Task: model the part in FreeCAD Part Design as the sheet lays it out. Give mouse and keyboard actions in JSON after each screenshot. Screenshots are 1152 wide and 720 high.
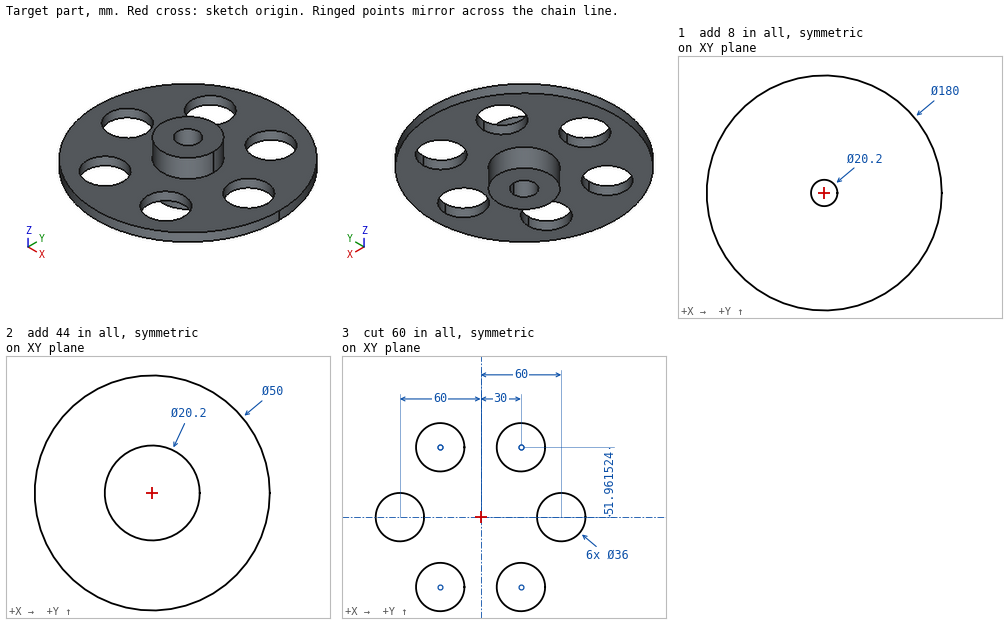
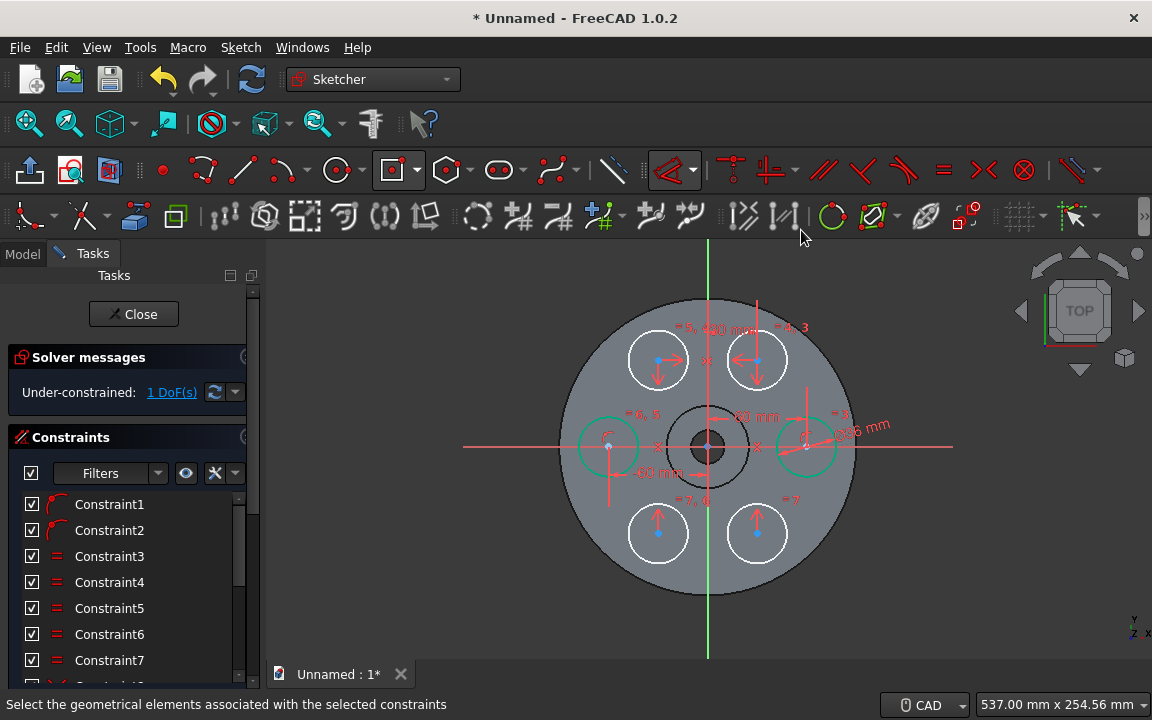
{"action": "left_click", "coordinate": [757, 360]}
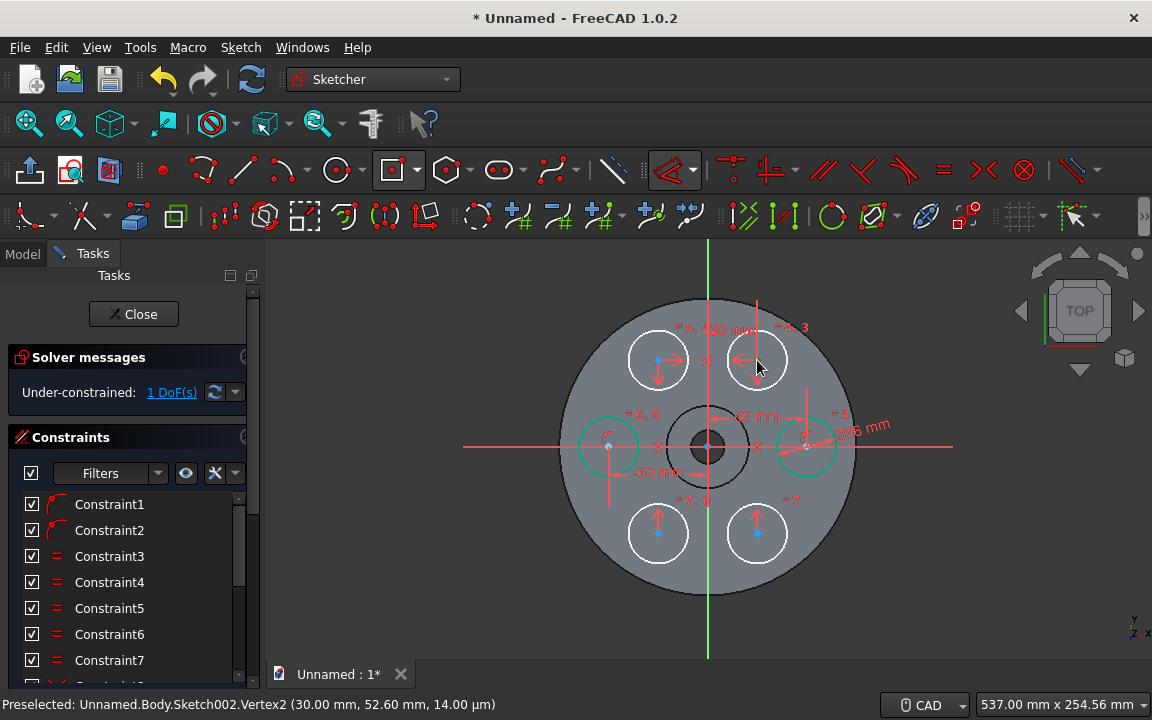
{"action": "key", "text": "i"}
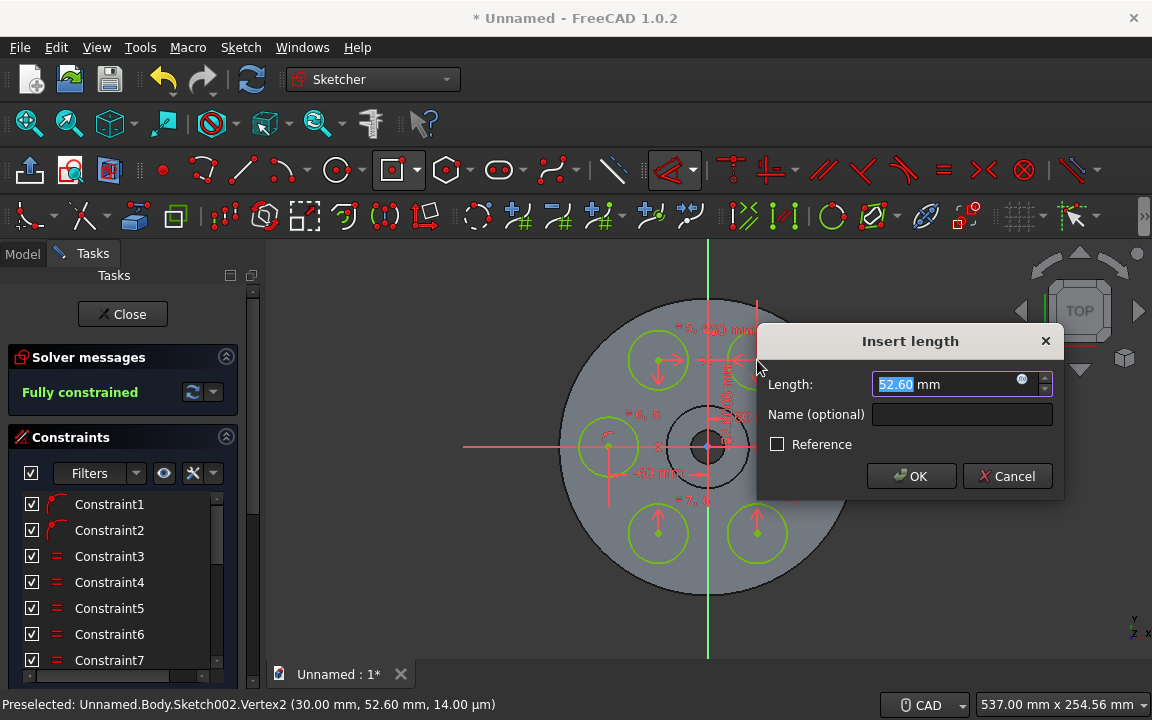
{"action": "type", "text": "51.961524"}
{"action": "key", "text": "Return"}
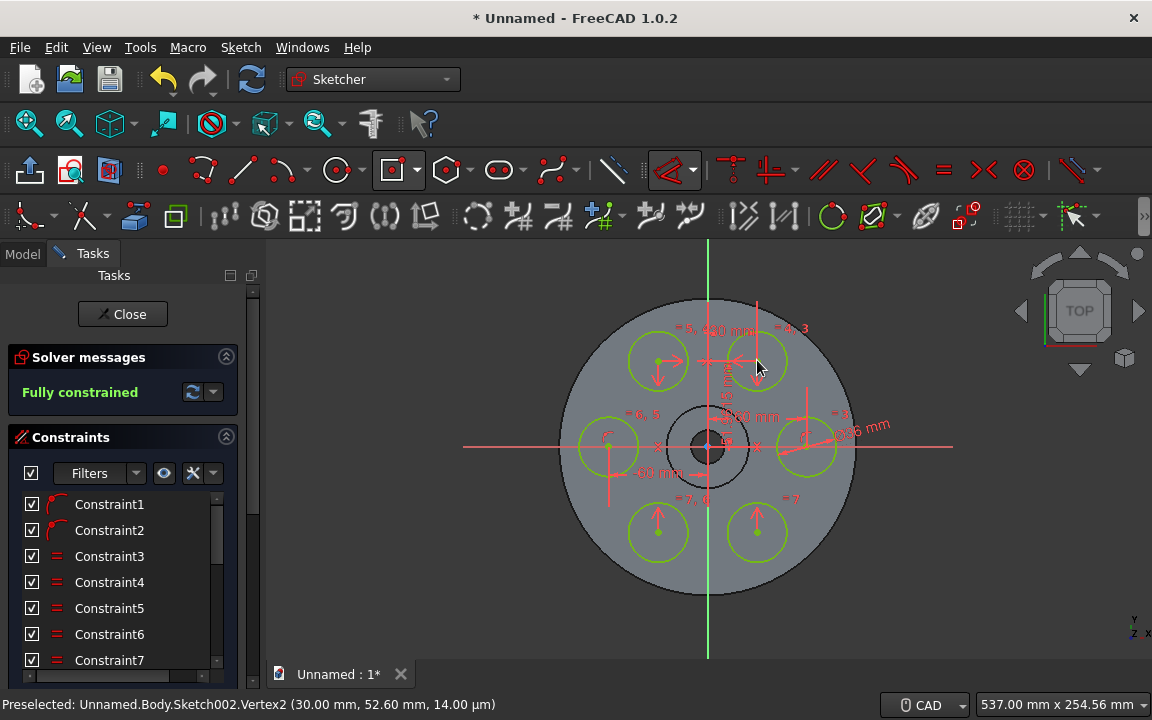
{"action": "left_click", "coordinate": [123, 314]}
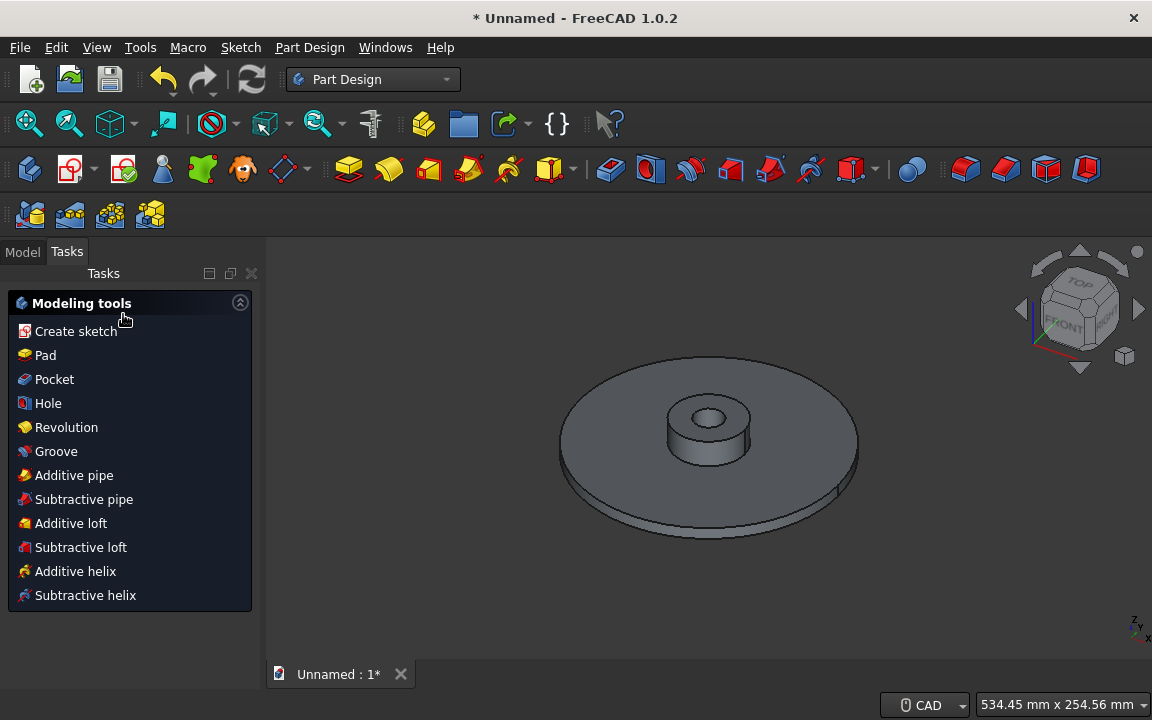
{"action": "left_click", "coordinate": [612, 170]}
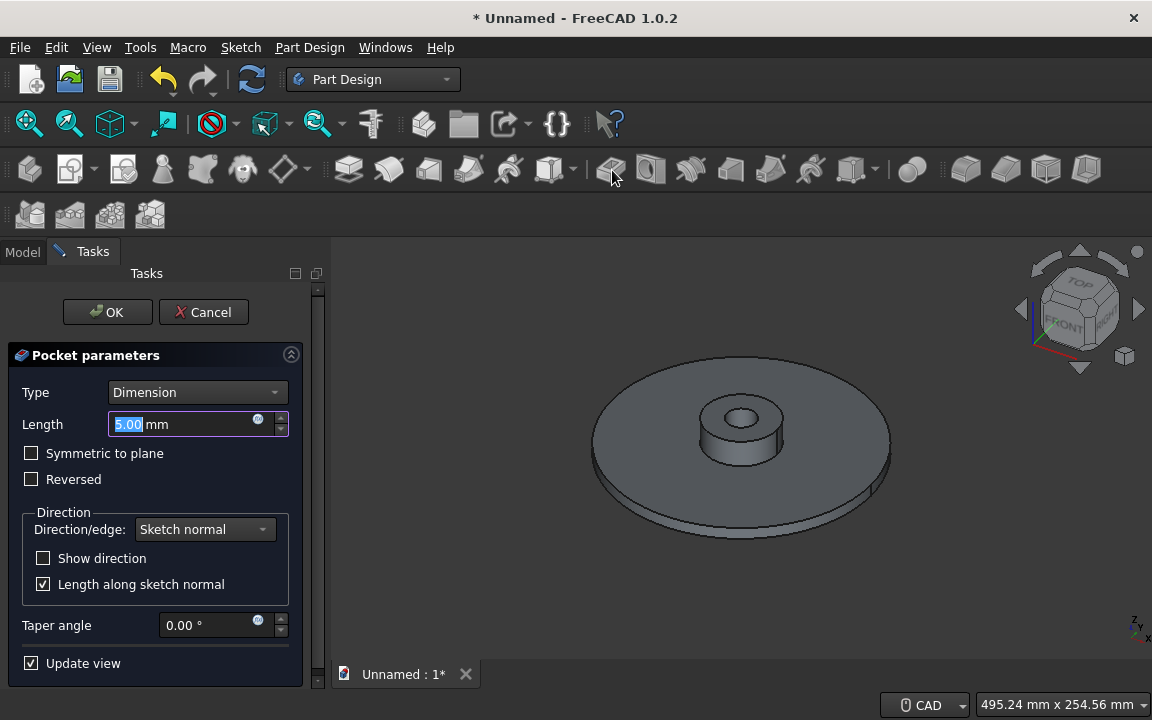
{"action": "type", "text": "60"}
{"action": "key", "text": "Tab"}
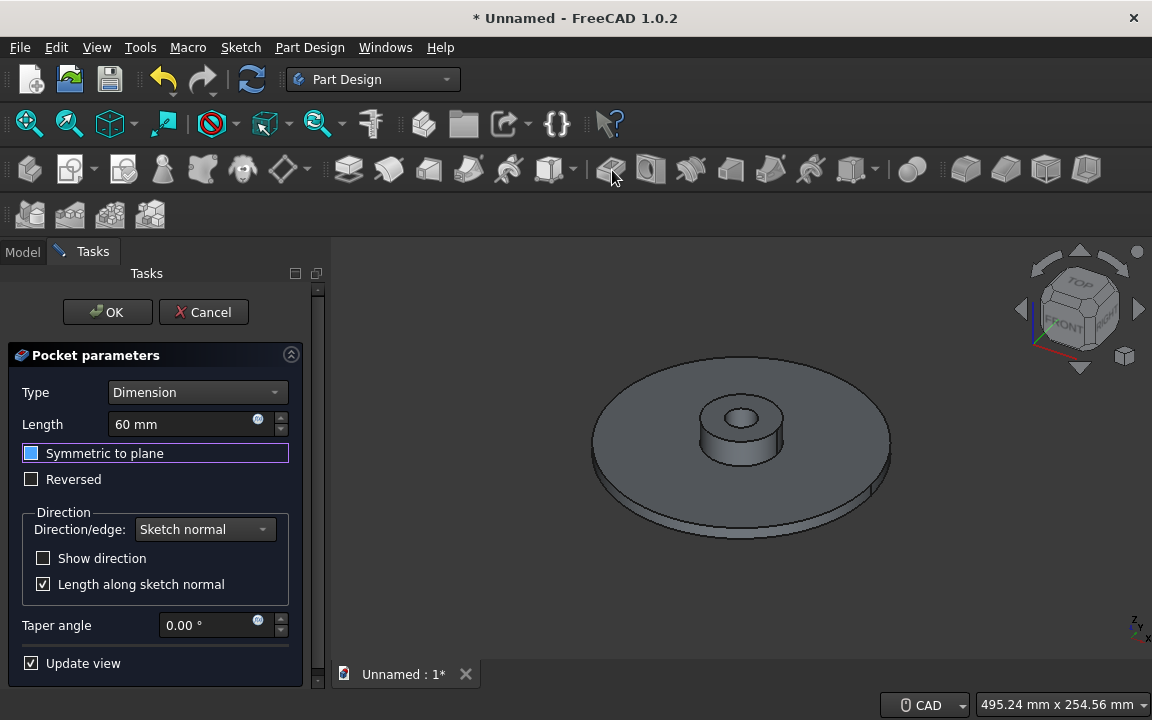
{"action": "left_click", "coordinate": [30, 453]}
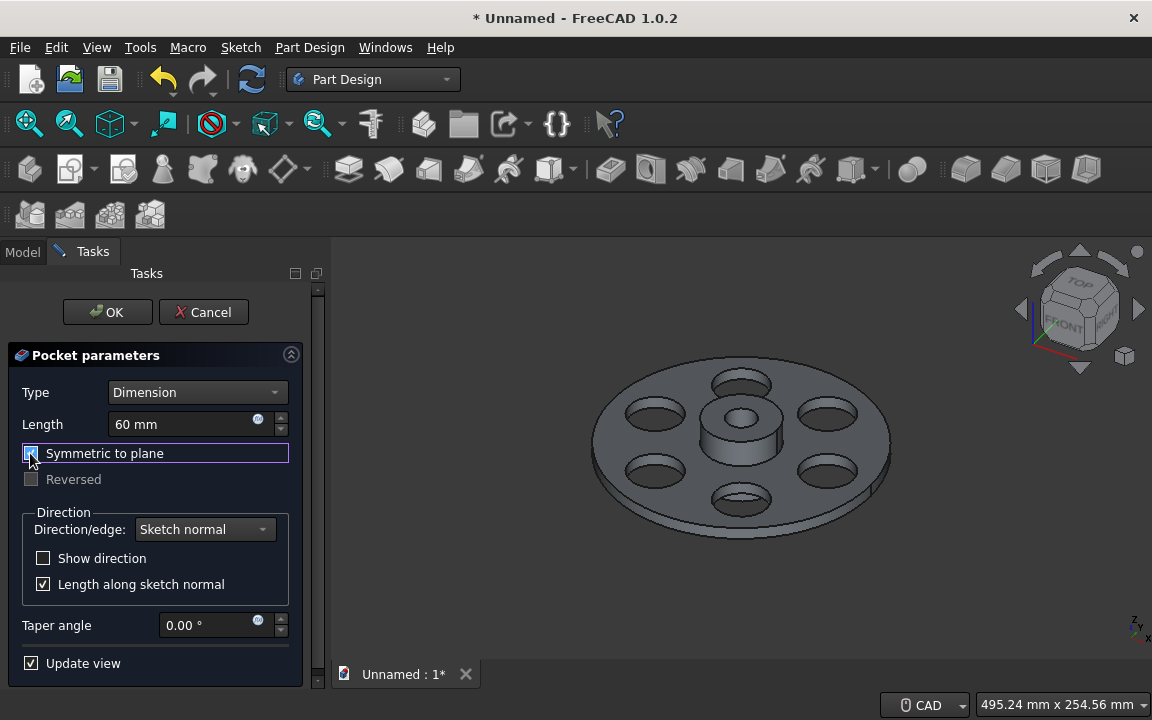
{"action": "left_click", "coordinate": [108, 312]}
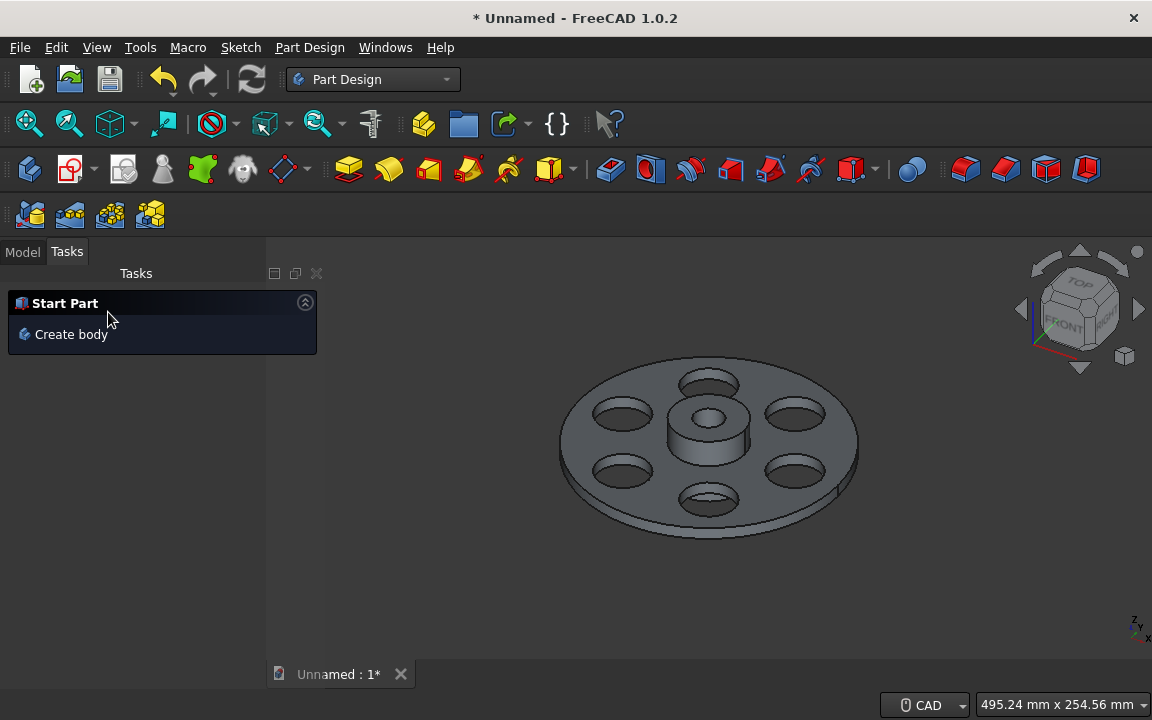
{"action": "key", "text": "0"}